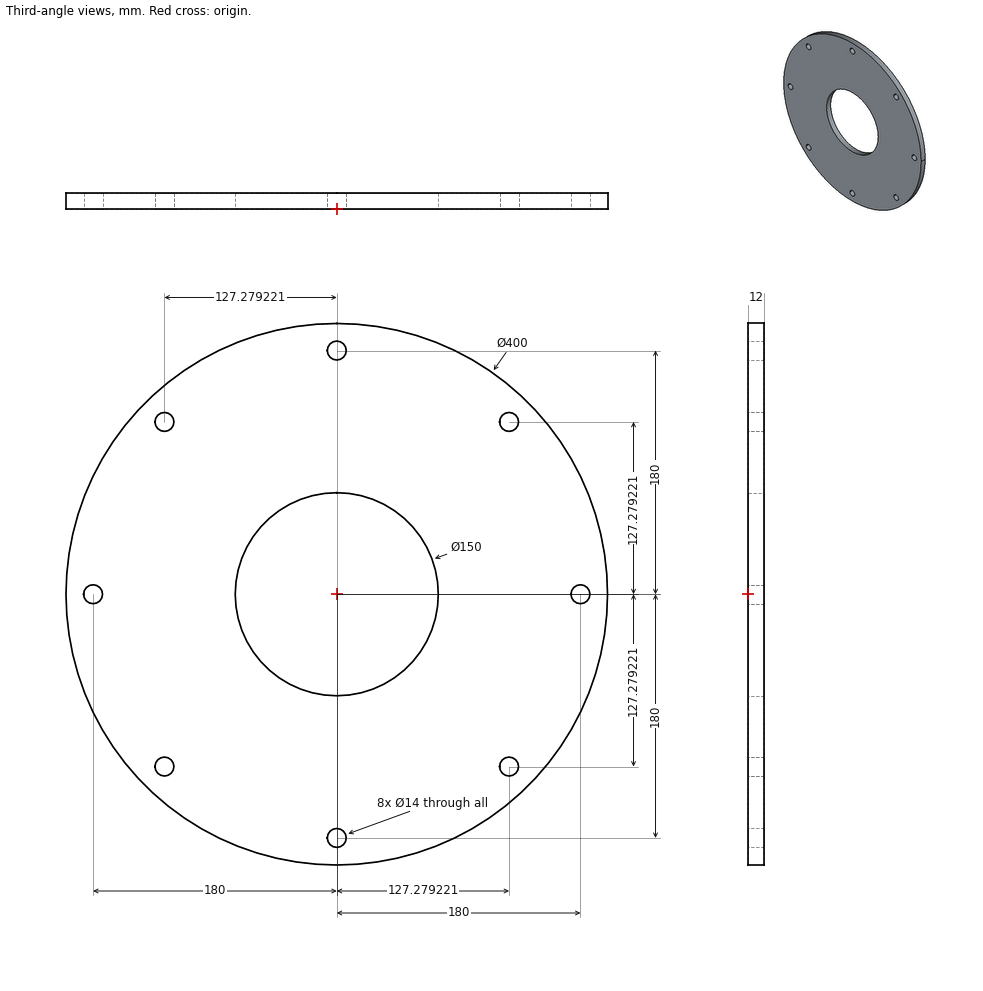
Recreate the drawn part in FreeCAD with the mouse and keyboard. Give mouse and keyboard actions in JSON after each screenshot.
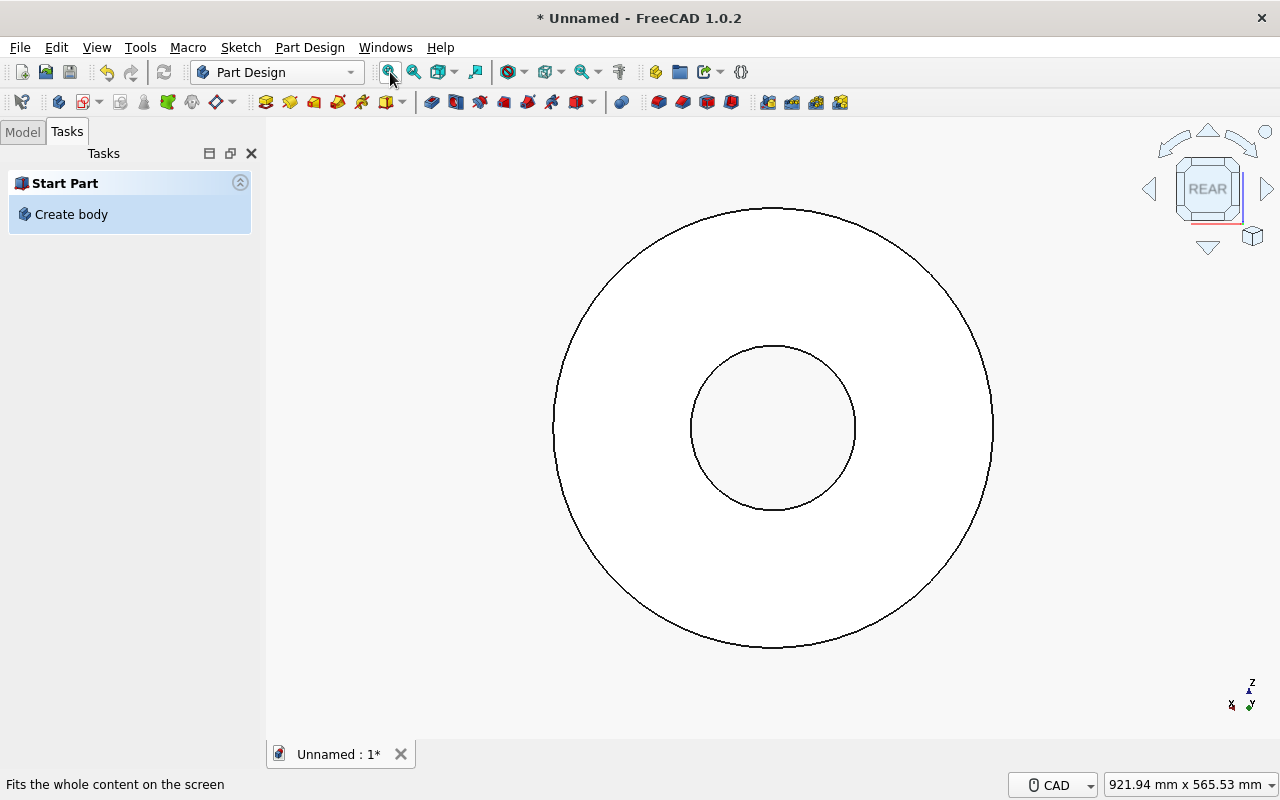
{"action": "left_click", "coordinate": [647, 364]}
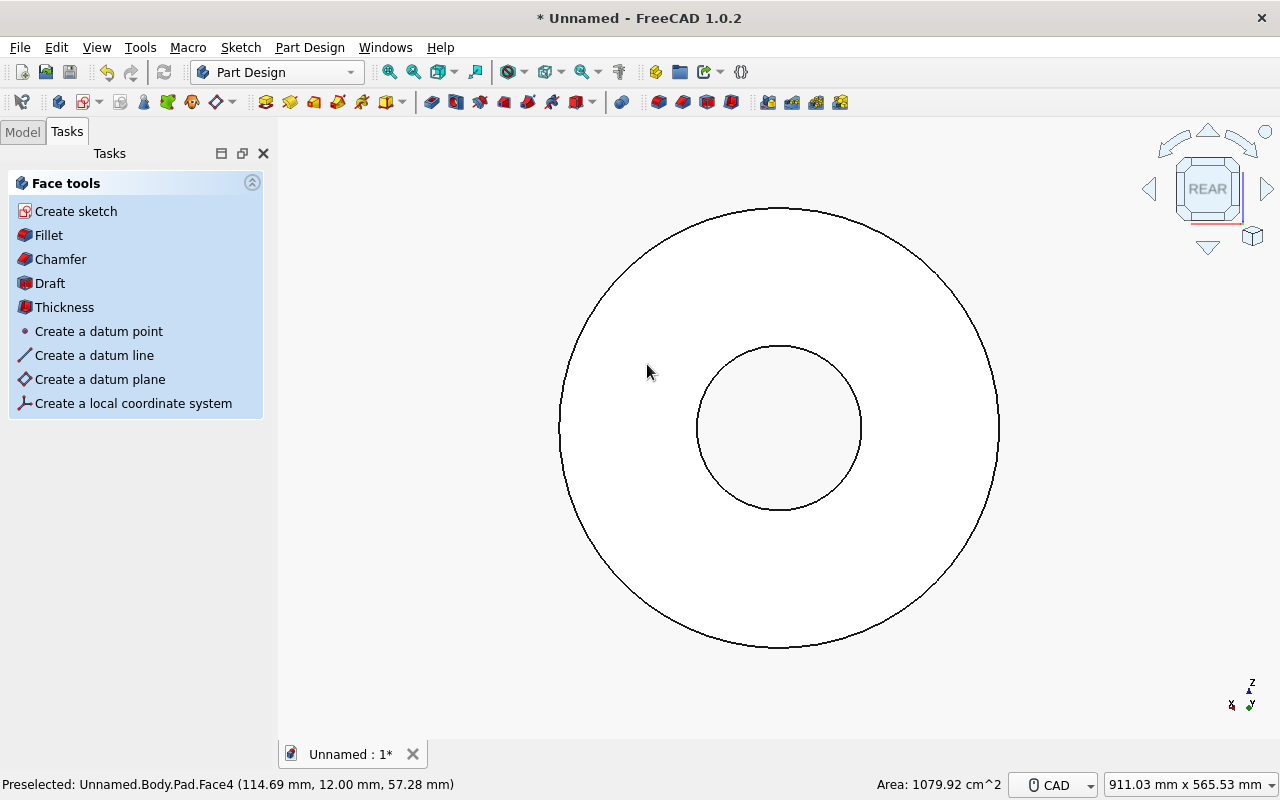
{"action": "left_click", "coordinate": [84, 102]}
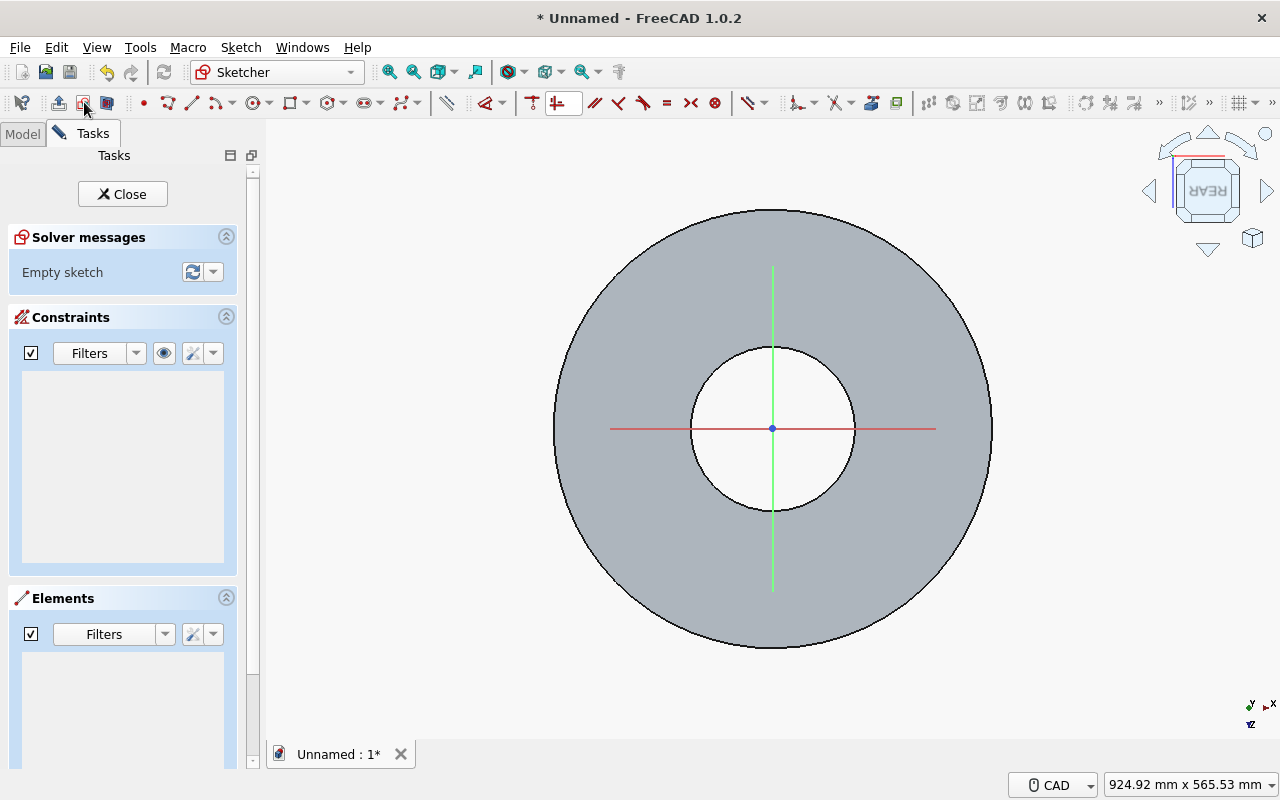
{"action": "left_click", "coordinate": [254, 104]}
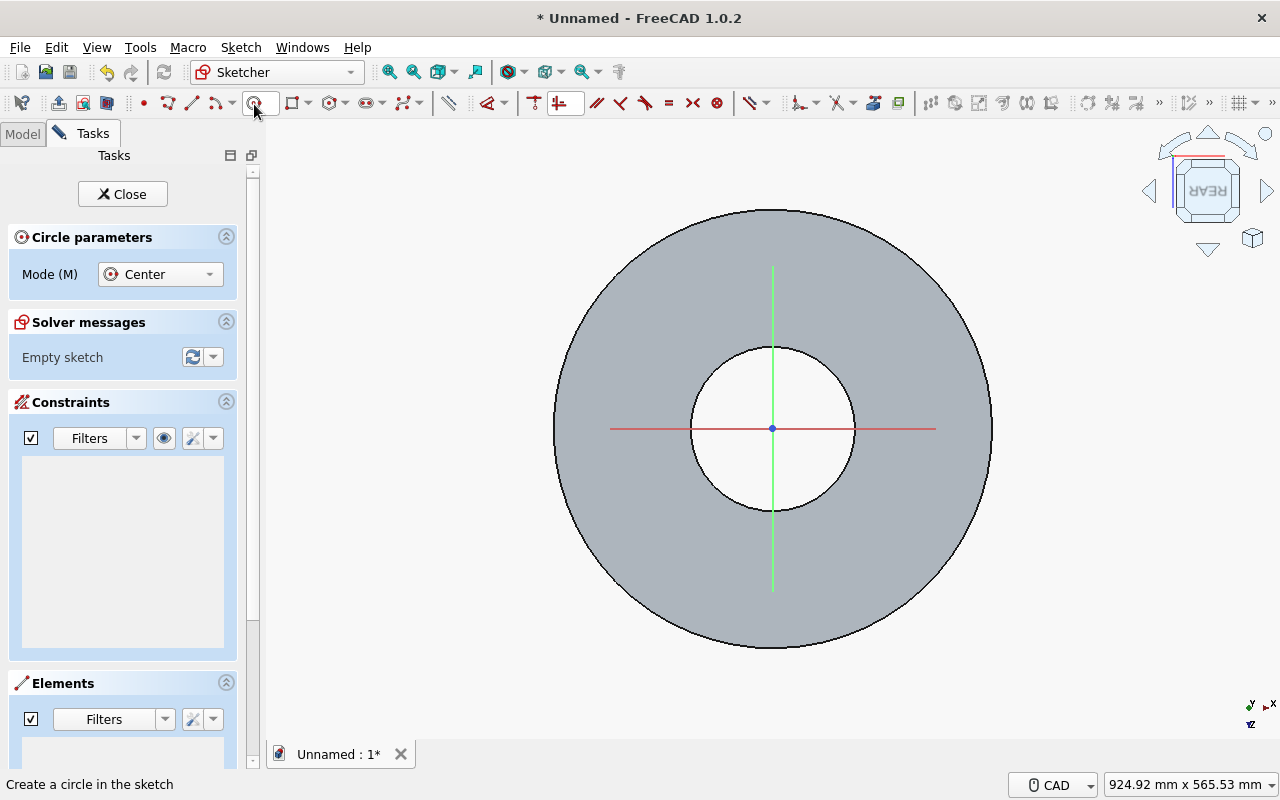
{"action": "scroll", "coordinate": [773, 232], "scroll_direction": "up", "scroll_amount": 6}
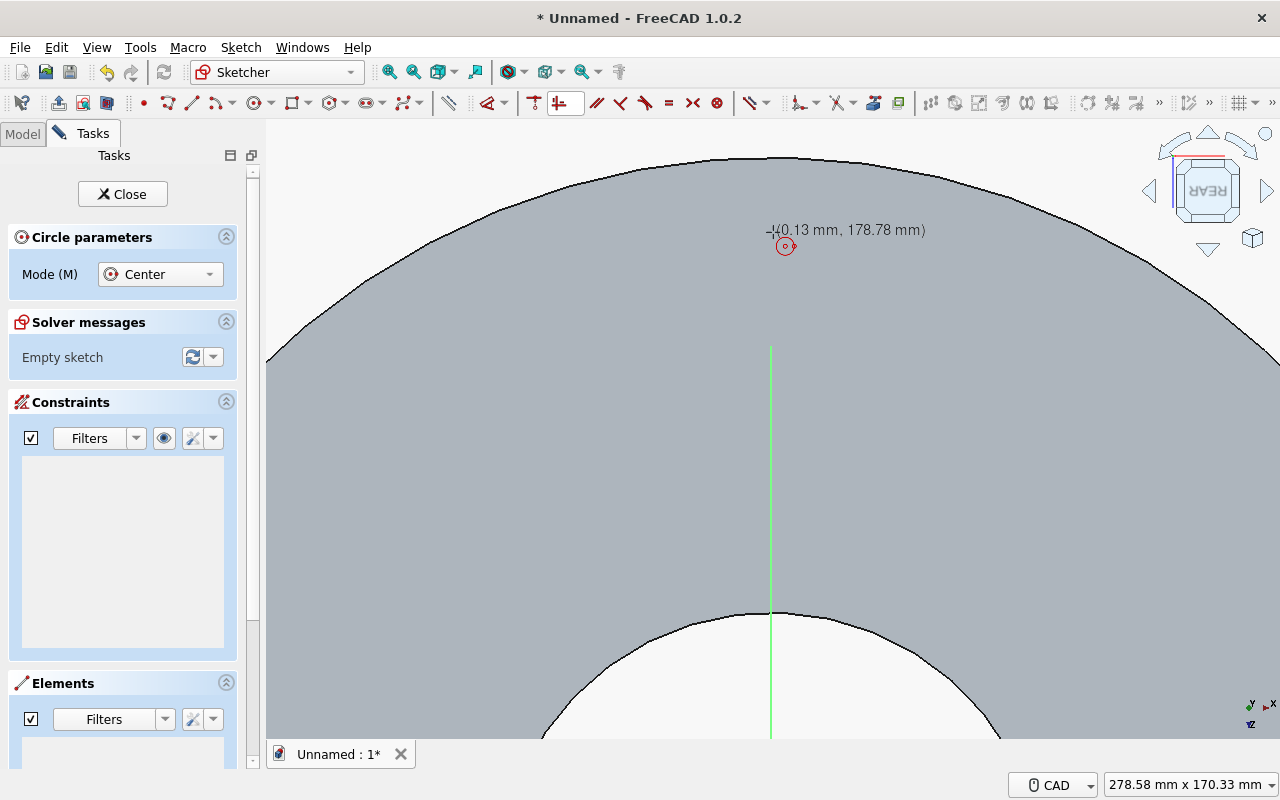
{"action": "left_click", "coordinate": [771, 230]}
{"action": "left_click", "coordinate": [789, 212]}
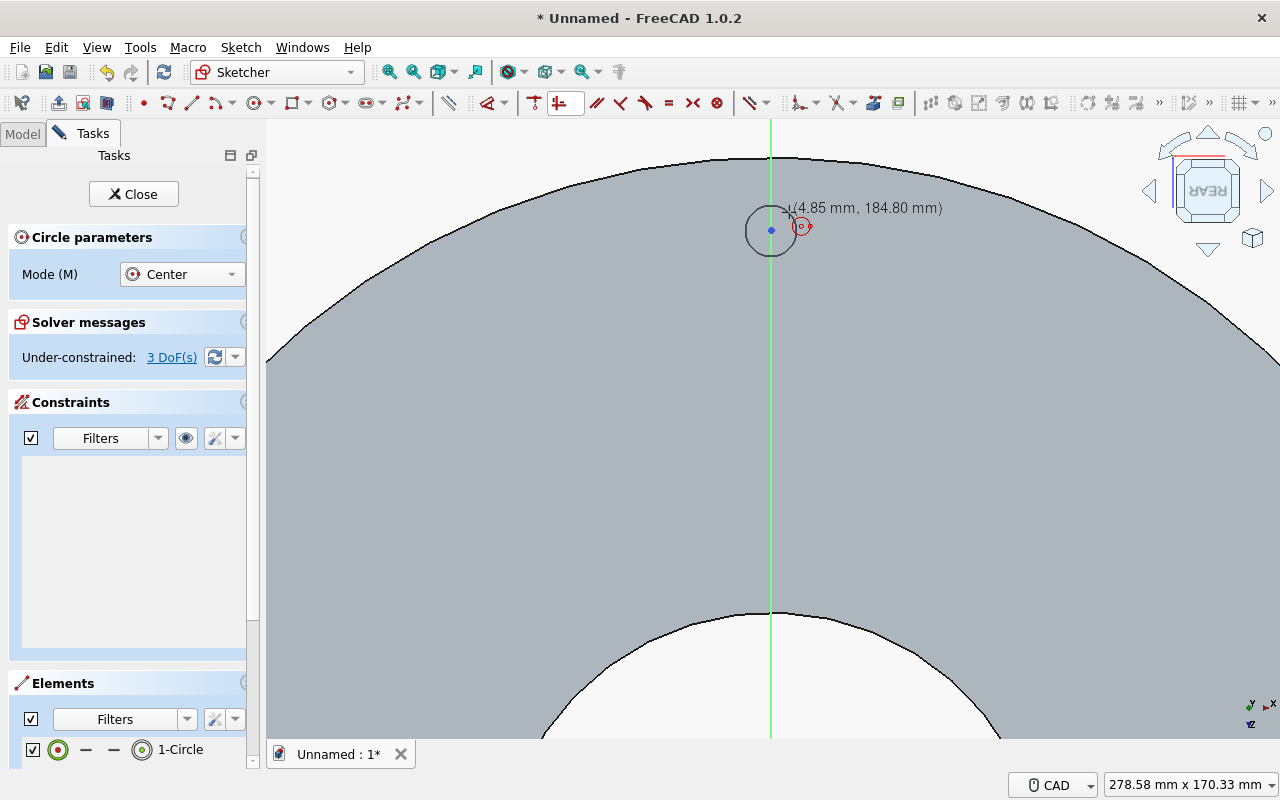
{"action": "scroll", "coordinate": [676, 232], "scroll_direction": "down", "scroll_amount": 6}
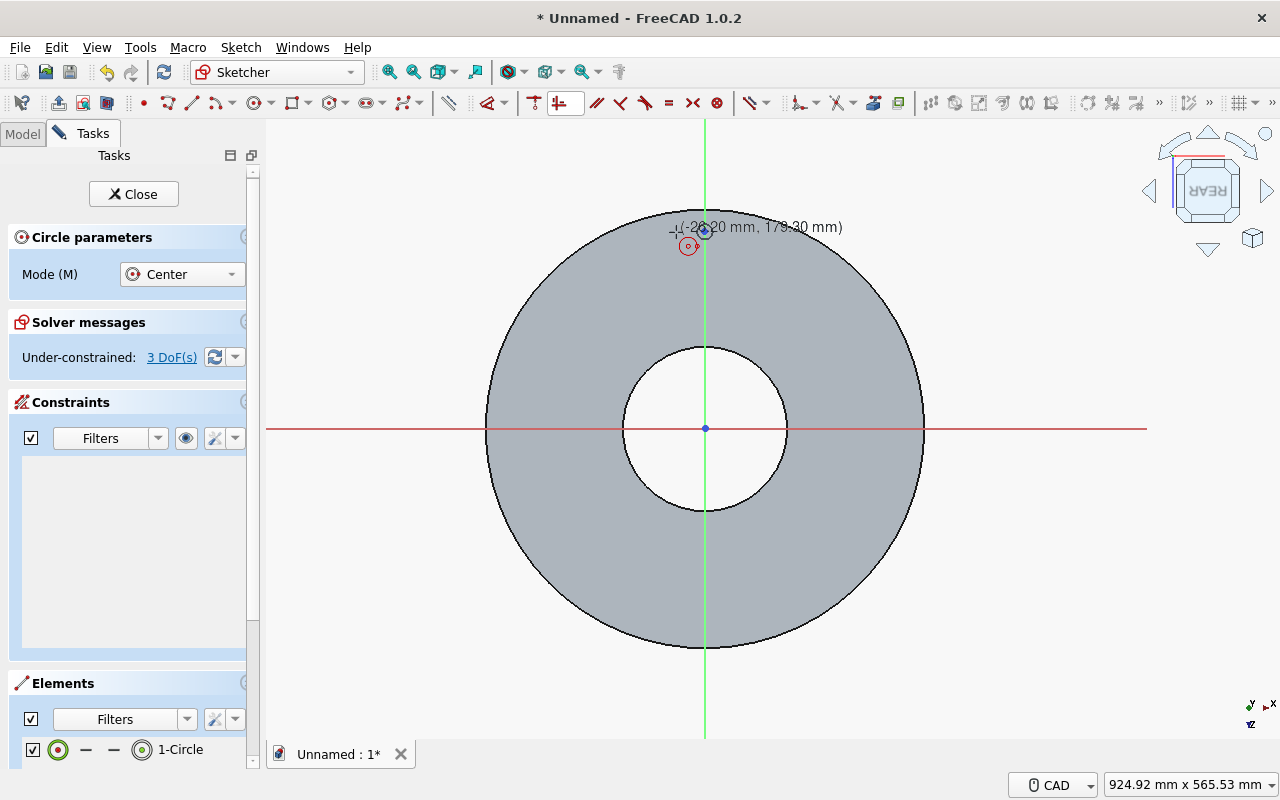
{"action": "scroll", "coordinate": [845, 289], "scroll_direction": "up", "scroll_amount": 6}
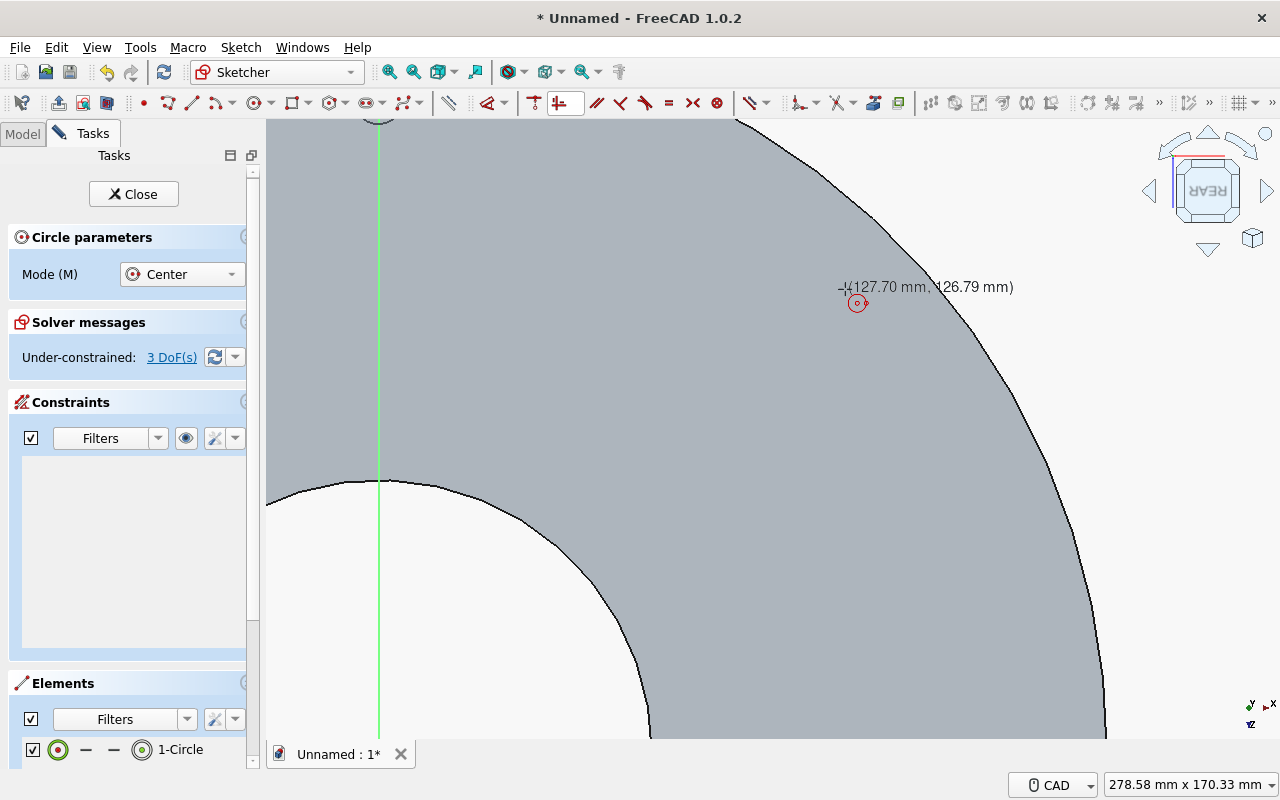
{"action": "left_click", "coordinate": [842, 290]}
{"action": "left_click", "coordinate": [860, 272]}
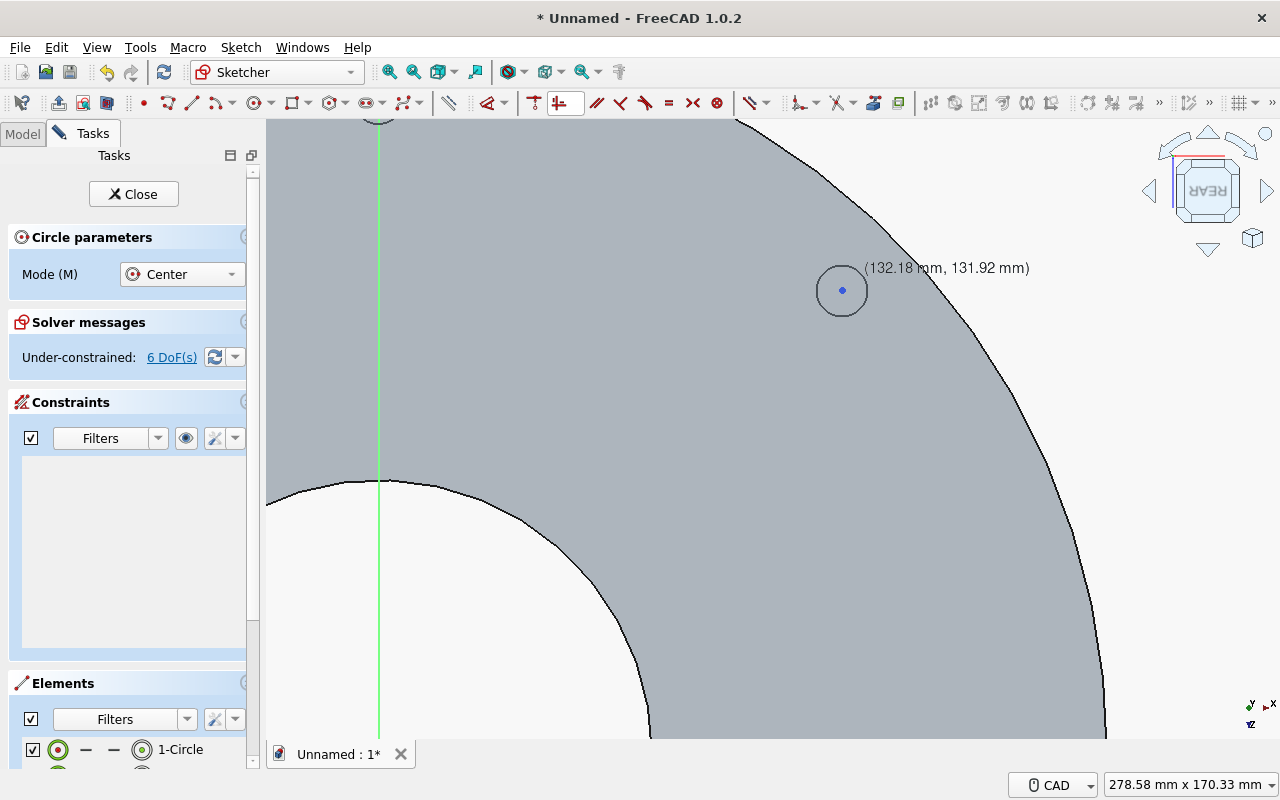
{"action": "scroll", "coordinate": [845, 289], "scroll_direction": "down", "scroll_amount": 6}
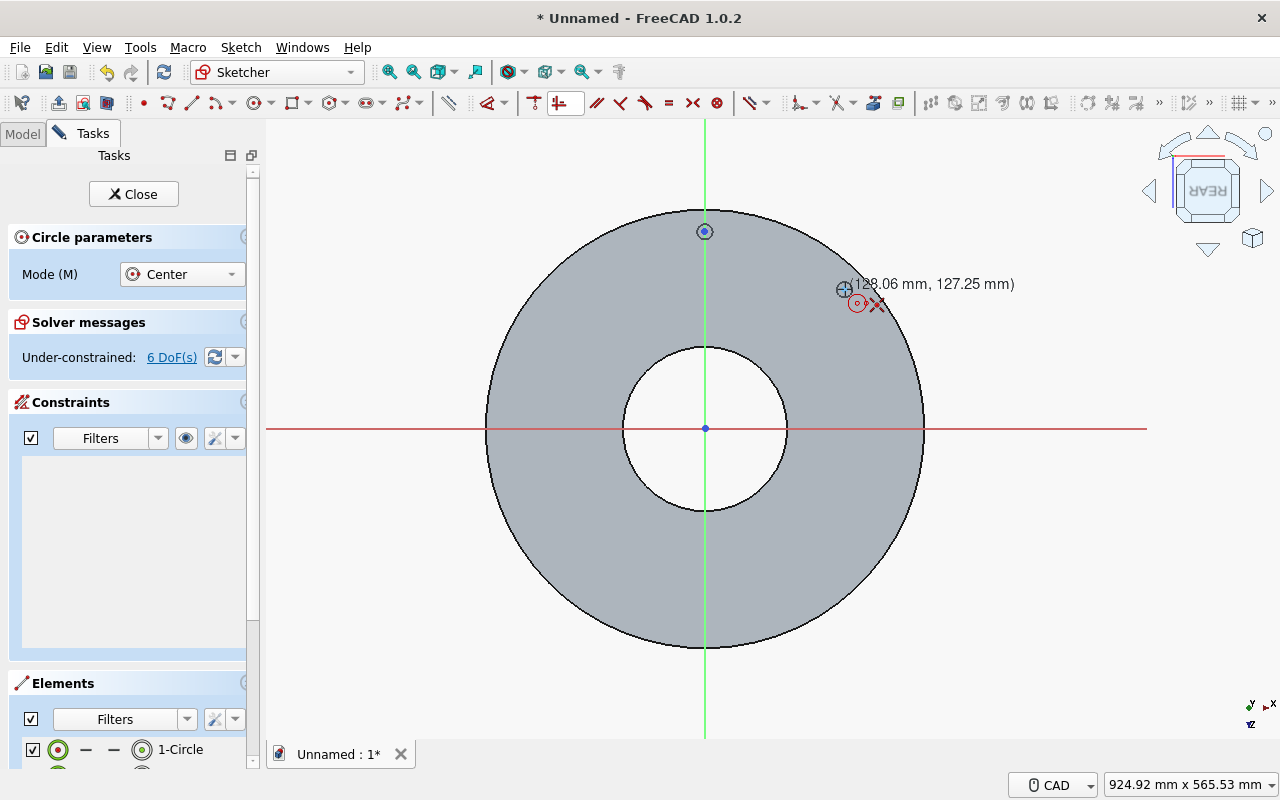
{"action": "scroll", "coordinate": [902, 429], "scroll_direction": "up", "scroll_amount": 6}